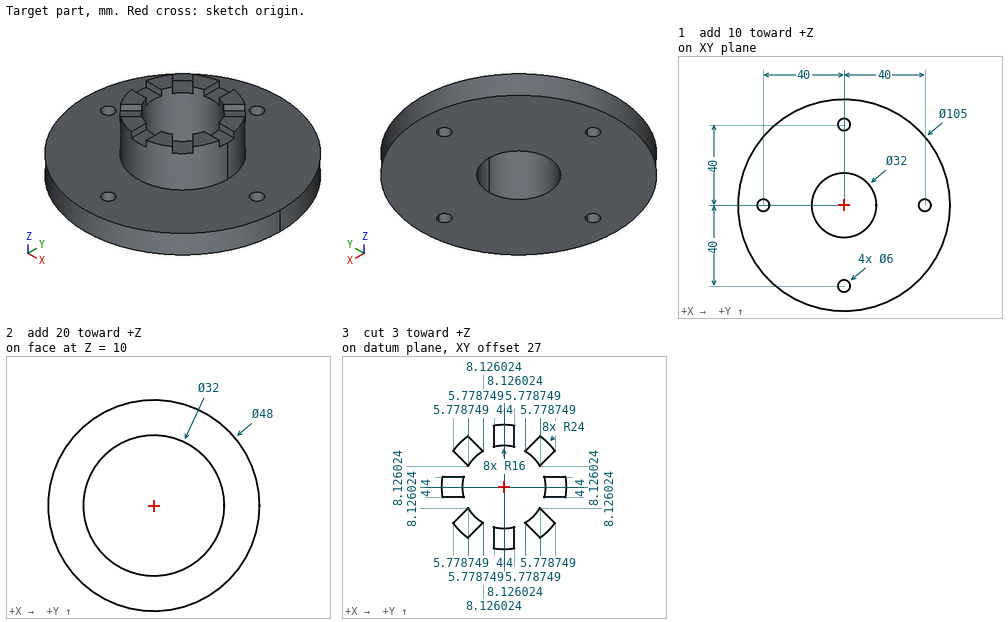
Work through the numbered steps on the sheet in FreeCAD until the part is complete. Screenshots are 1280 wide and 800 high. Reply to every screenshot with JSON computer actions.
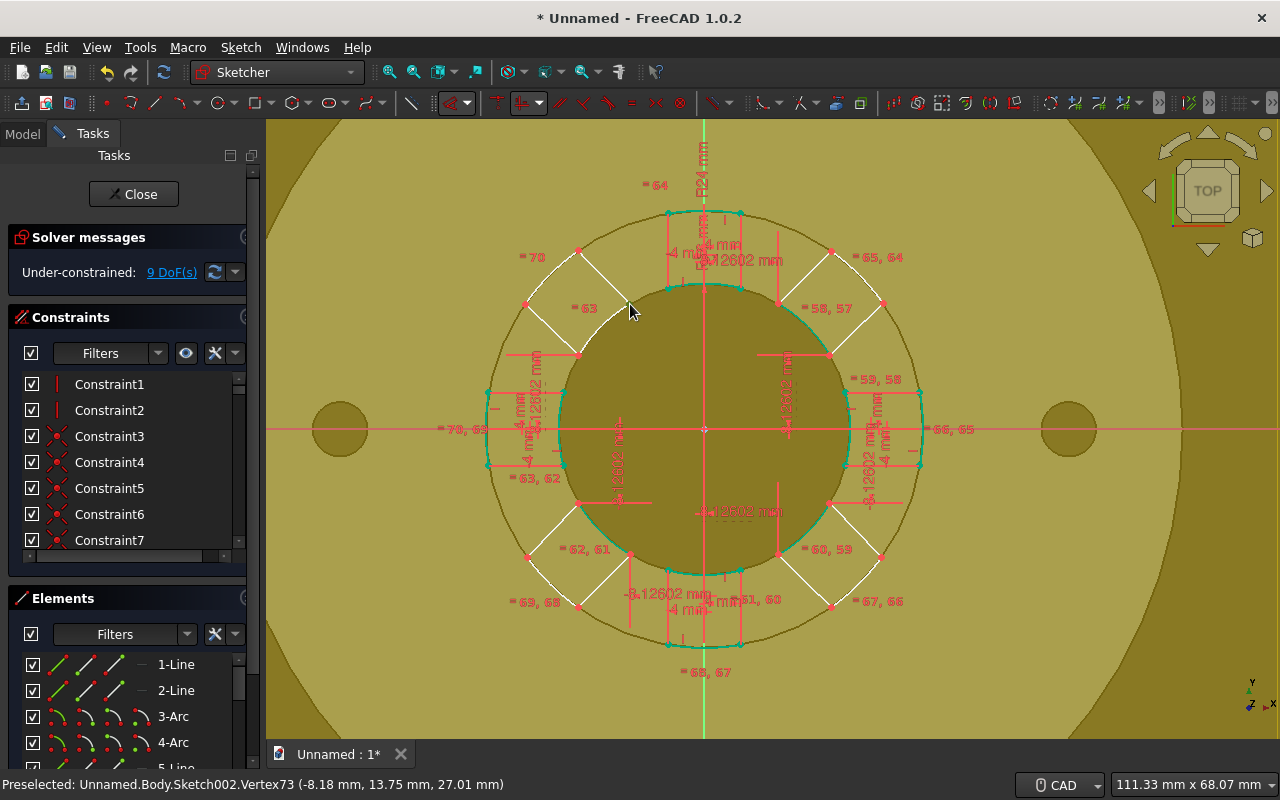
{"action": "left_click", "coordinate": [470, 104]}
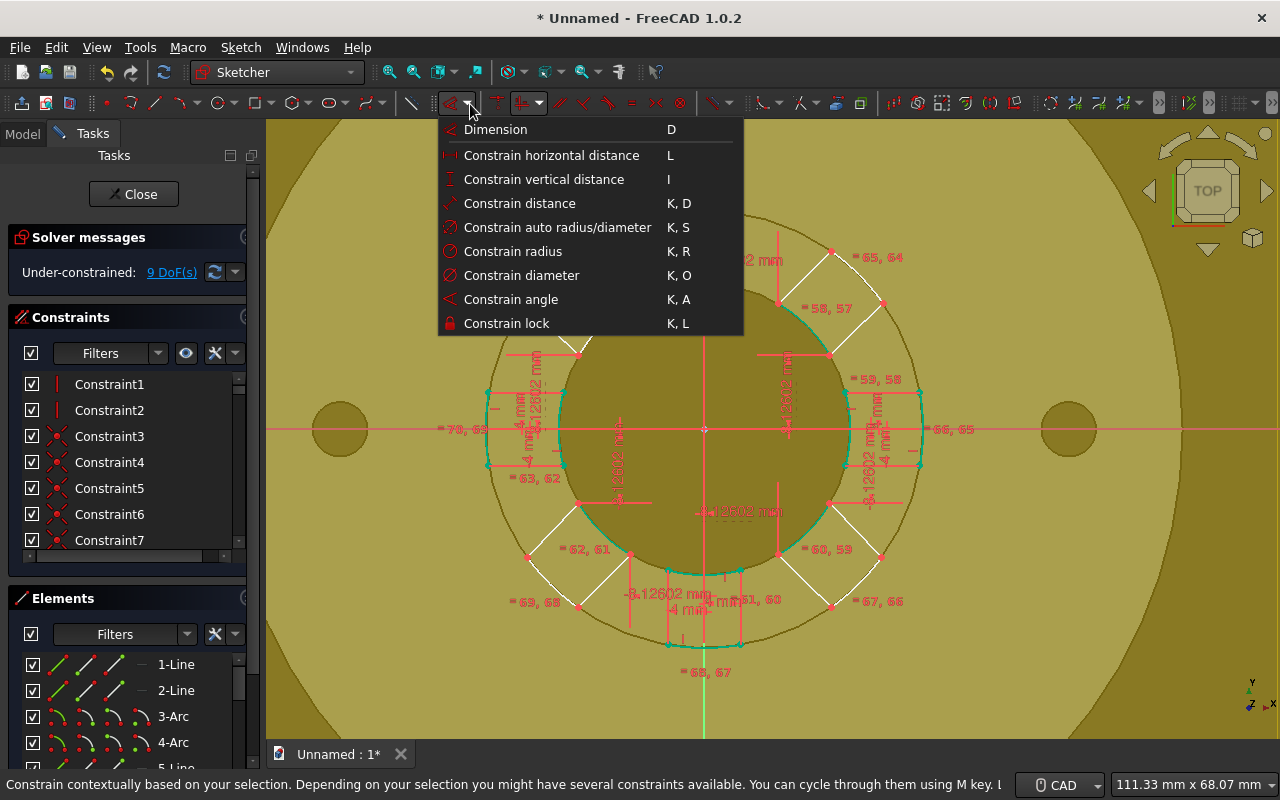
{"action": "left_click", "coordinate": [591, 155]}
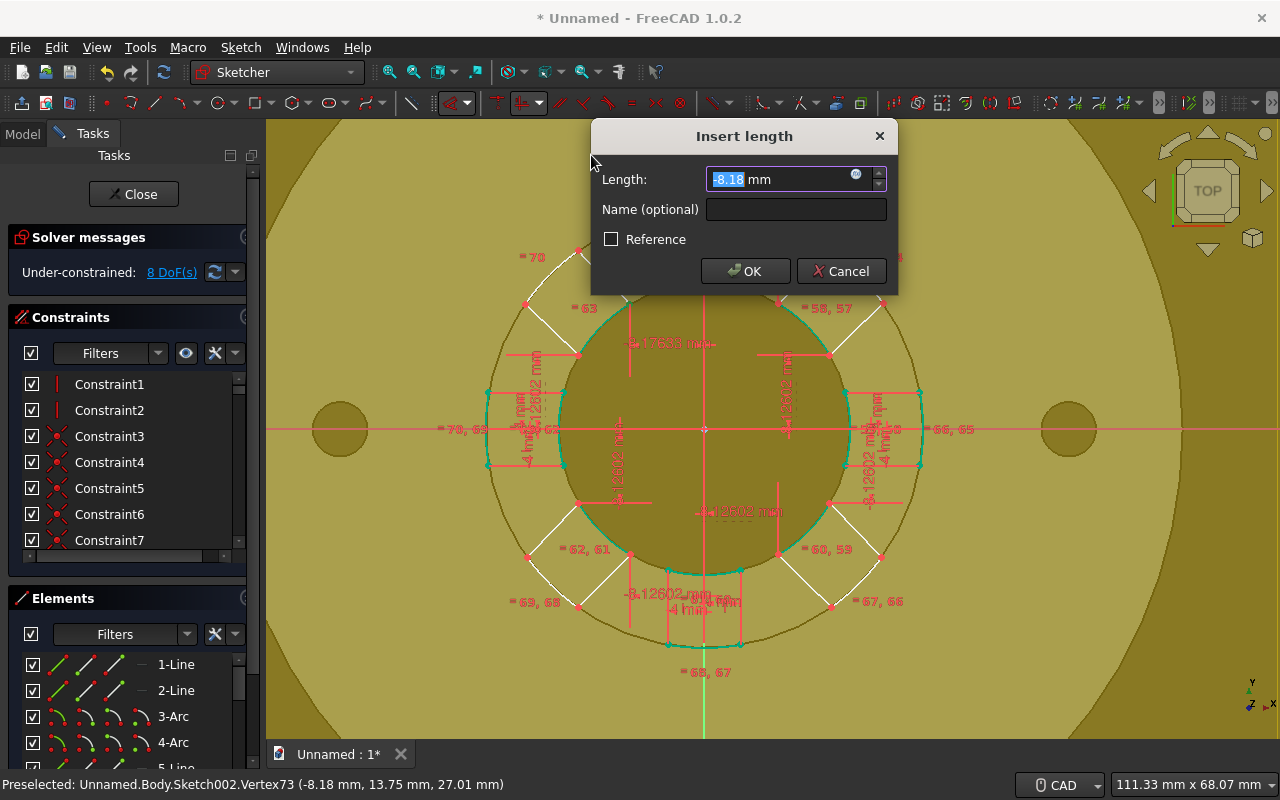
{"action": "type", "text": "-8.126024"}
{"action": "key", "text": "Return"}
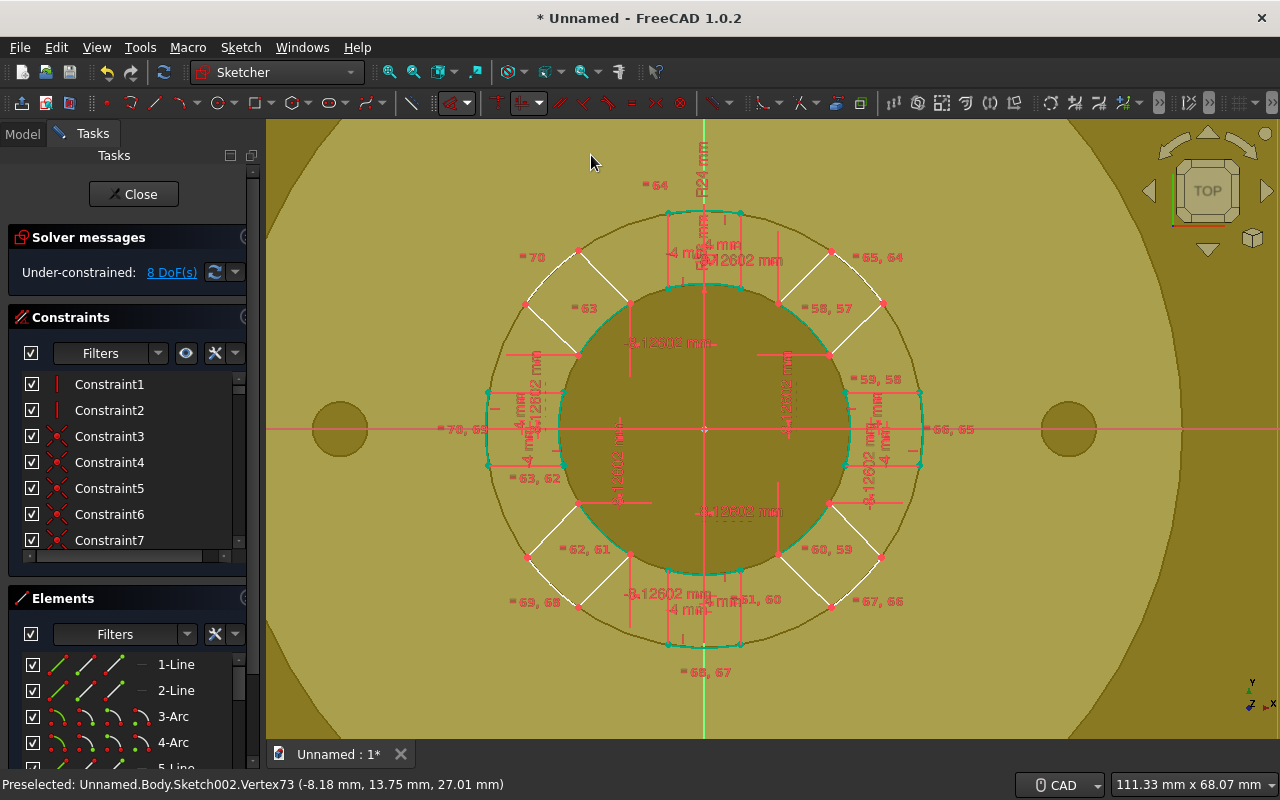
{"action": "left_click", "coordinate": [815, 267]}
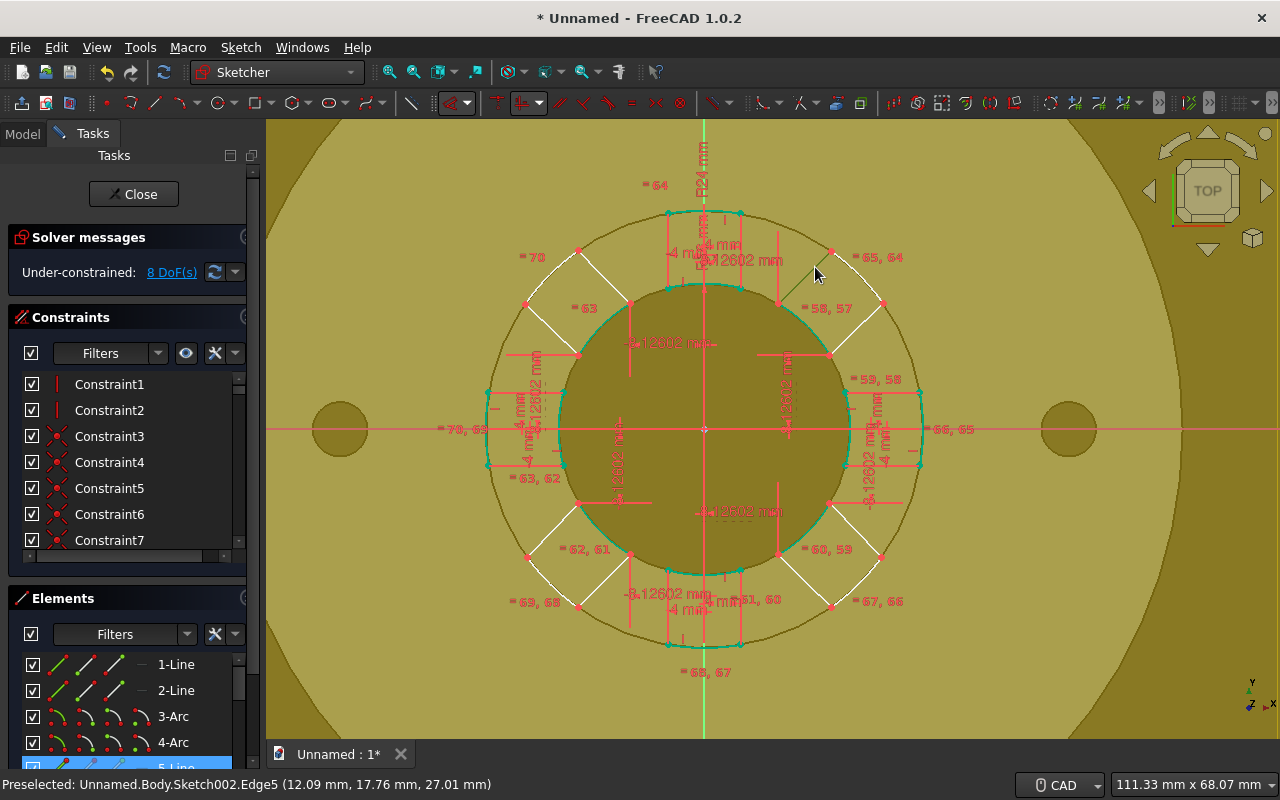
{"action": "left_click", "coordinate": [470, 104]}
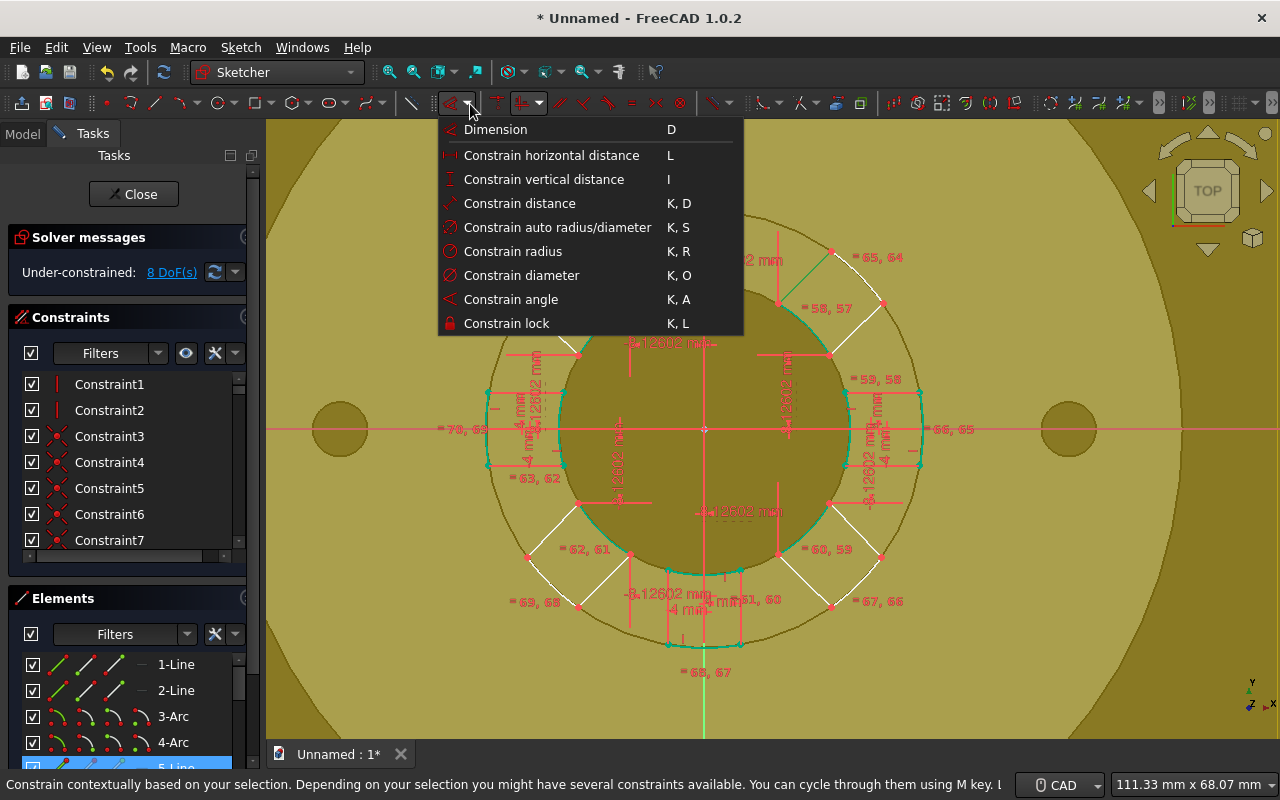
{"action": "left_click", "coordinate": [591, 155]}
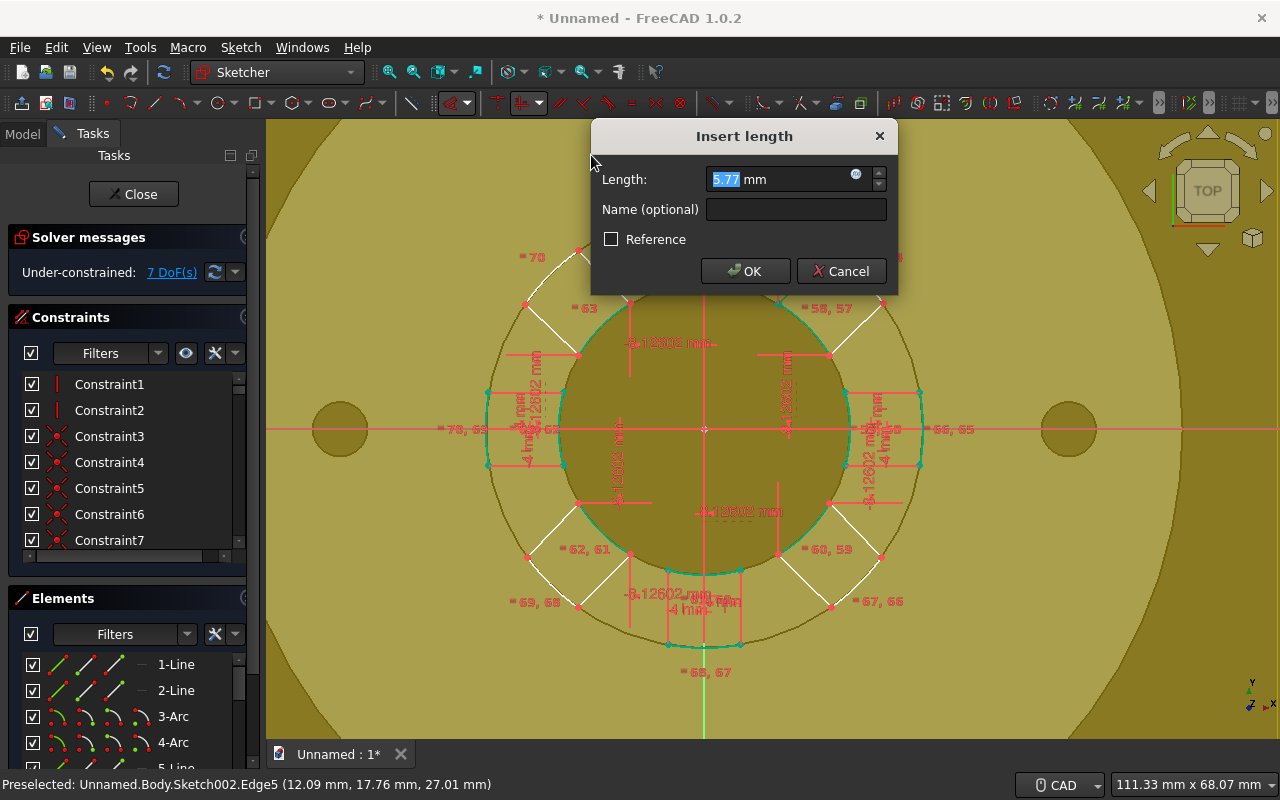
{"action": "type", "text": "5.778749"}
{"action": "key", "text": "Return"}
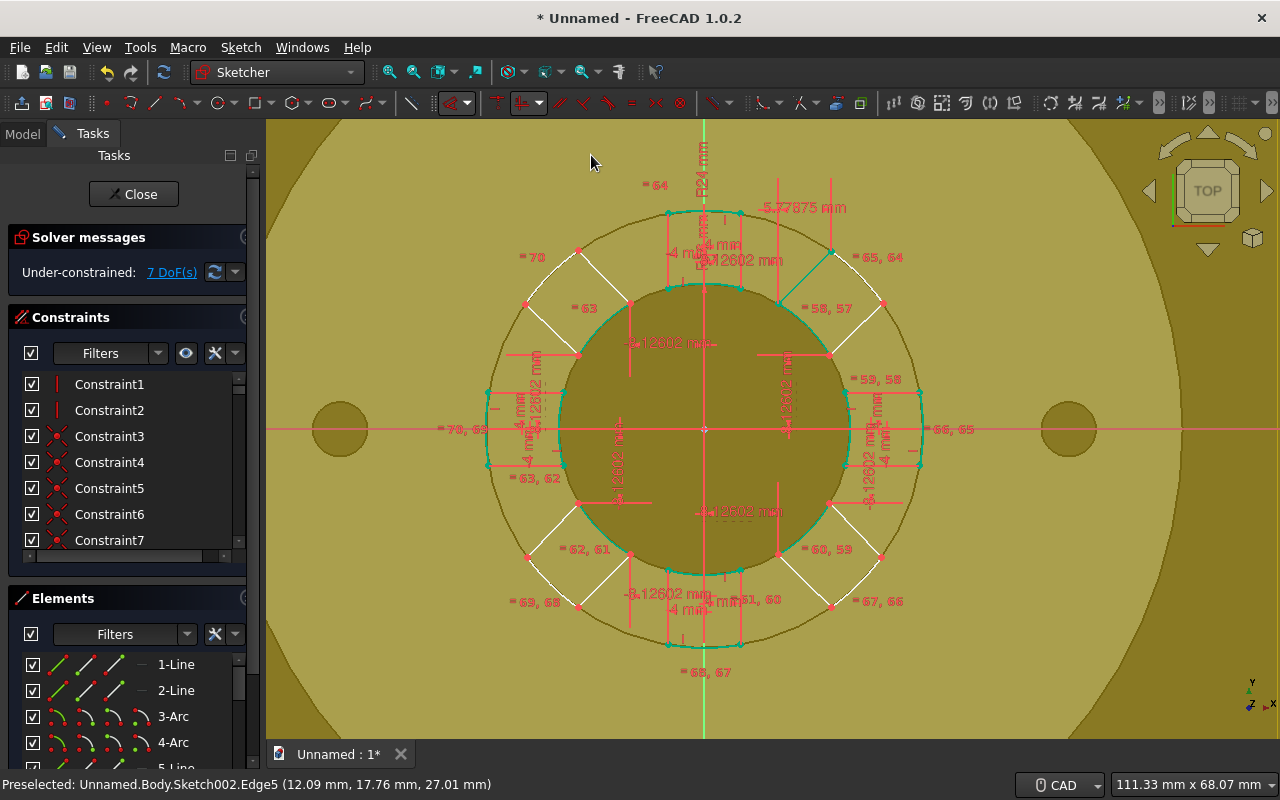
{"action": "left_click", "coordinate": [846, 340]}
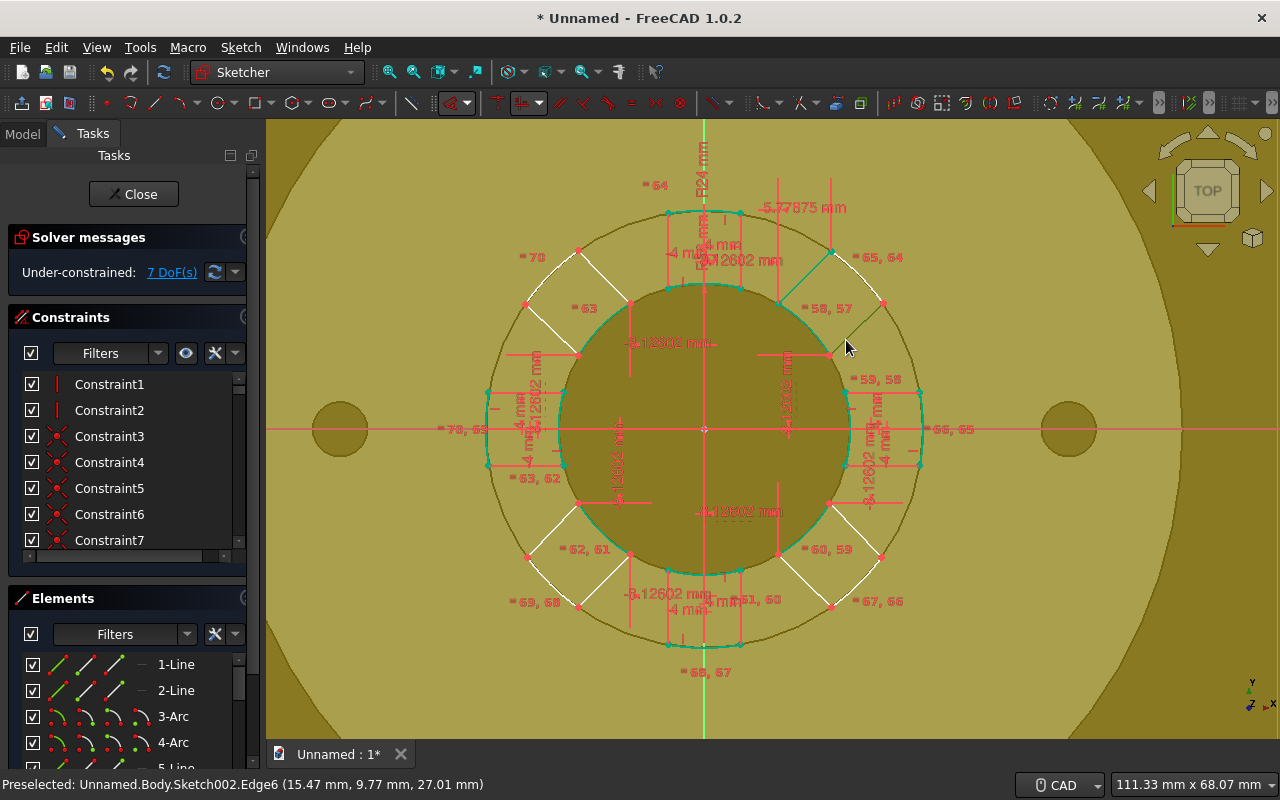
{"action": "key", "text": "l"}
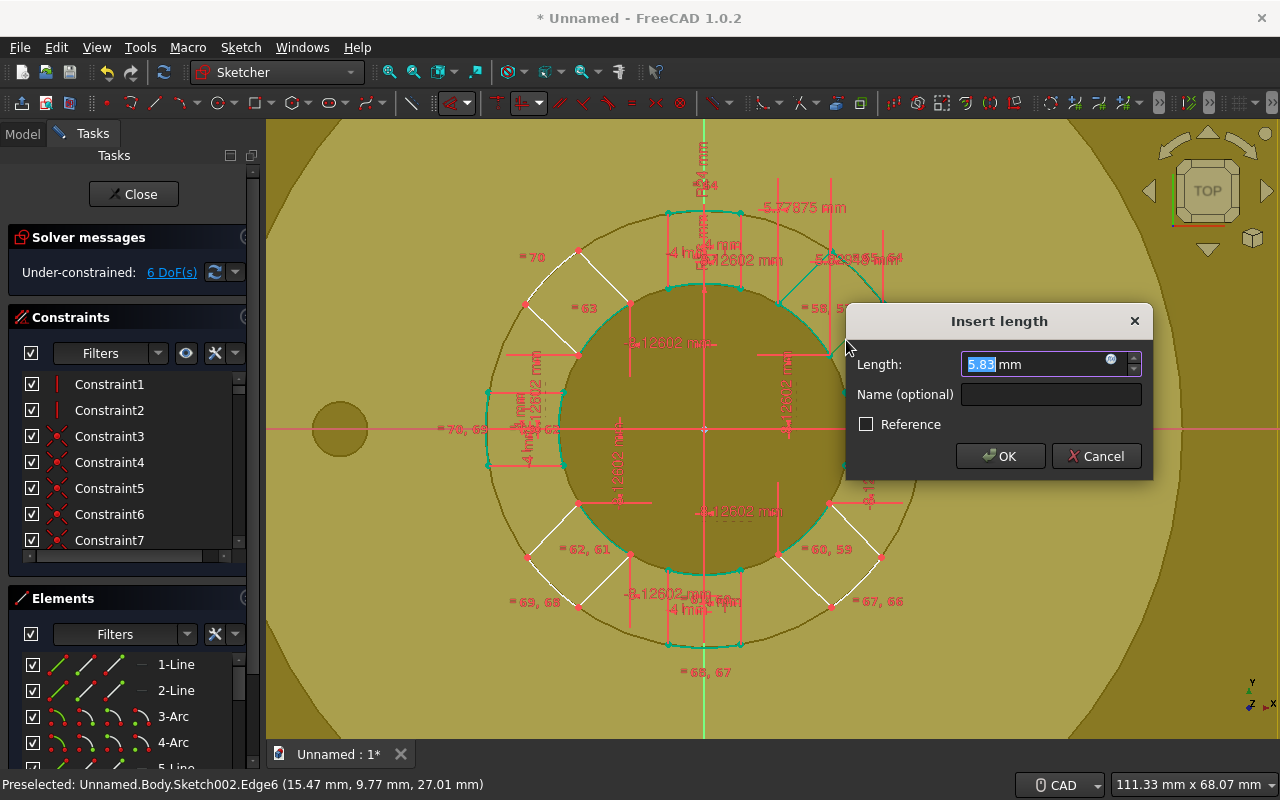
{"action": "type", "text": "5.778749"}
{"action": "key", "text": "Return"}